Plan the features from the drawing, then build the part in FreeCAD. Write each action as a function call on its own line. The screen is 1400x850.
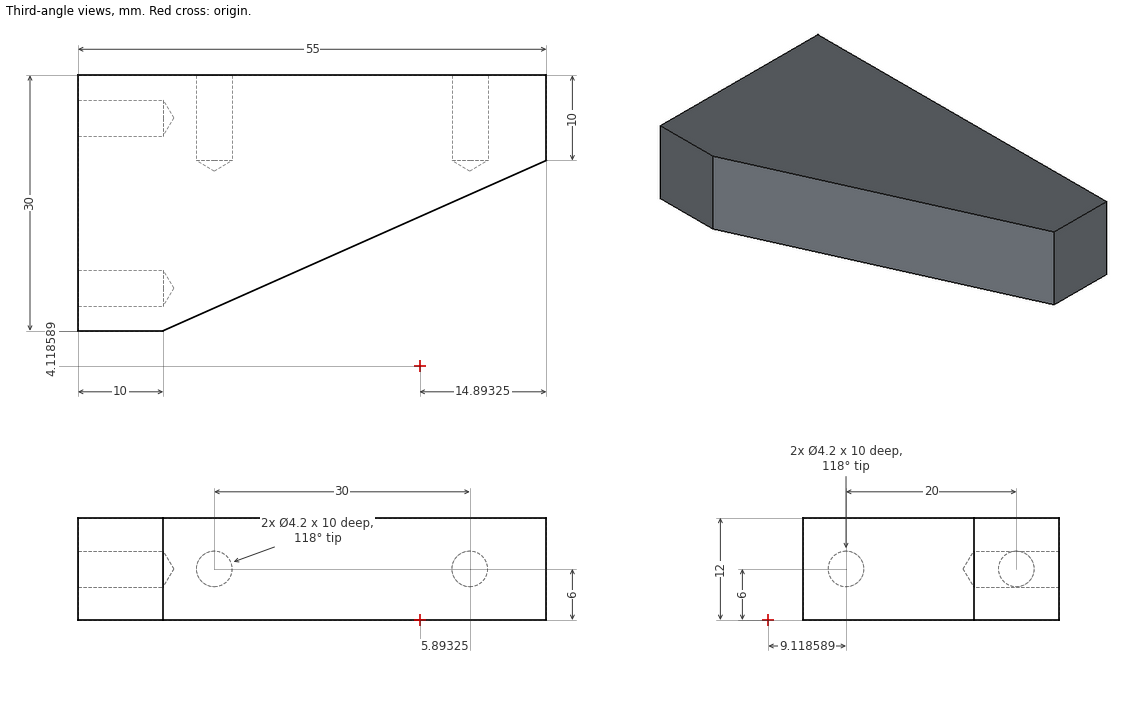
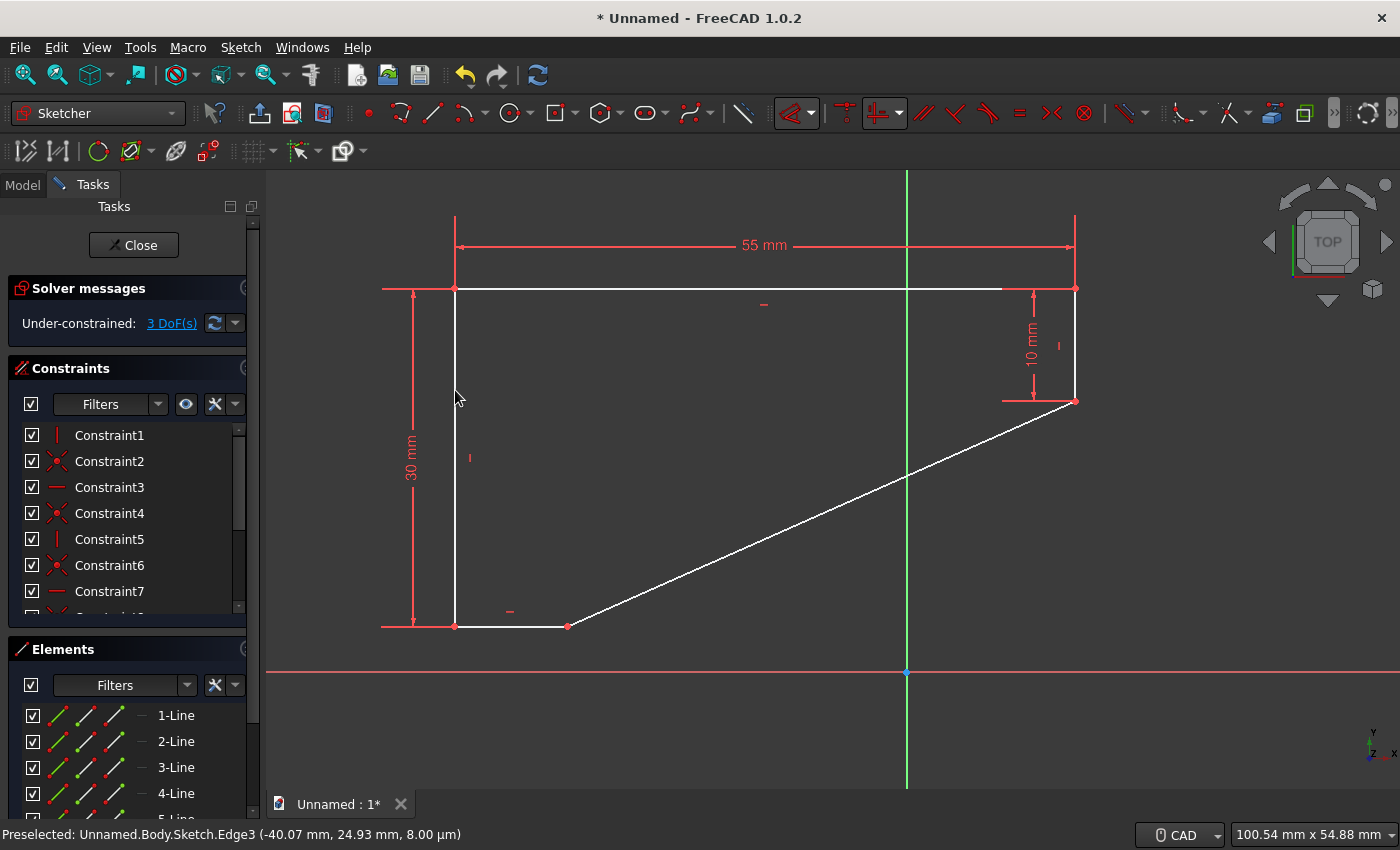
click(488, 627)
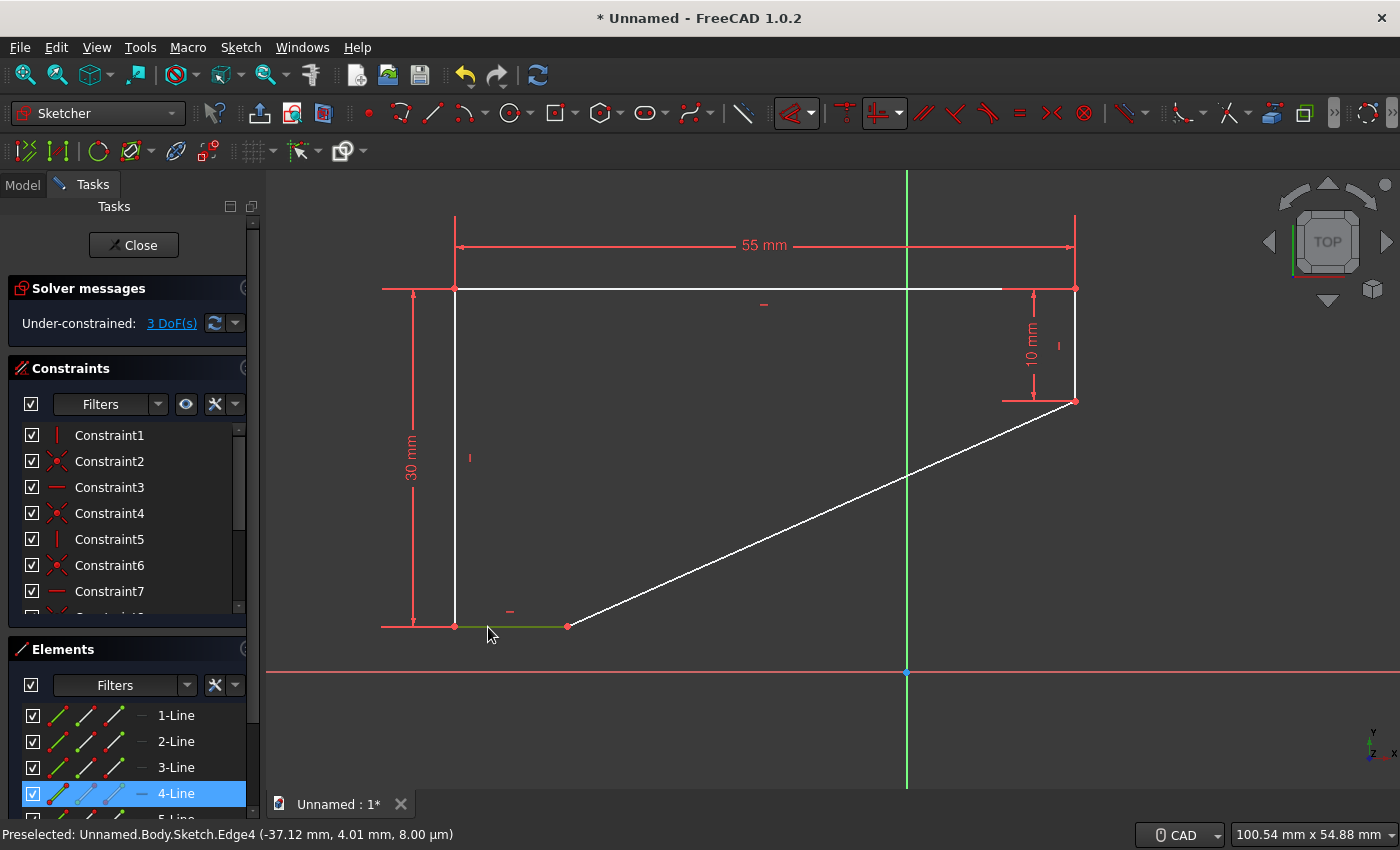
click(814, 114)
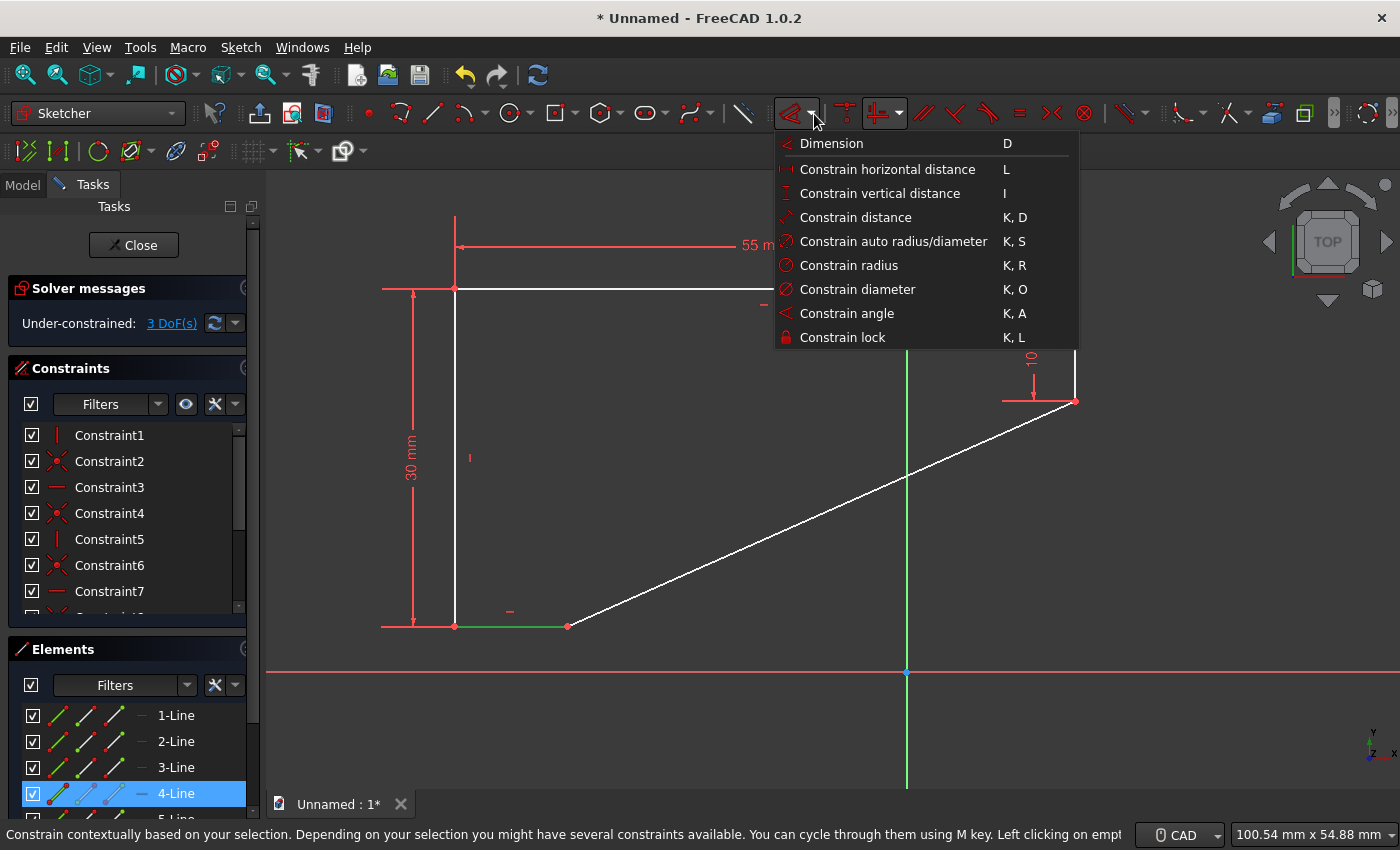
click(927, 169)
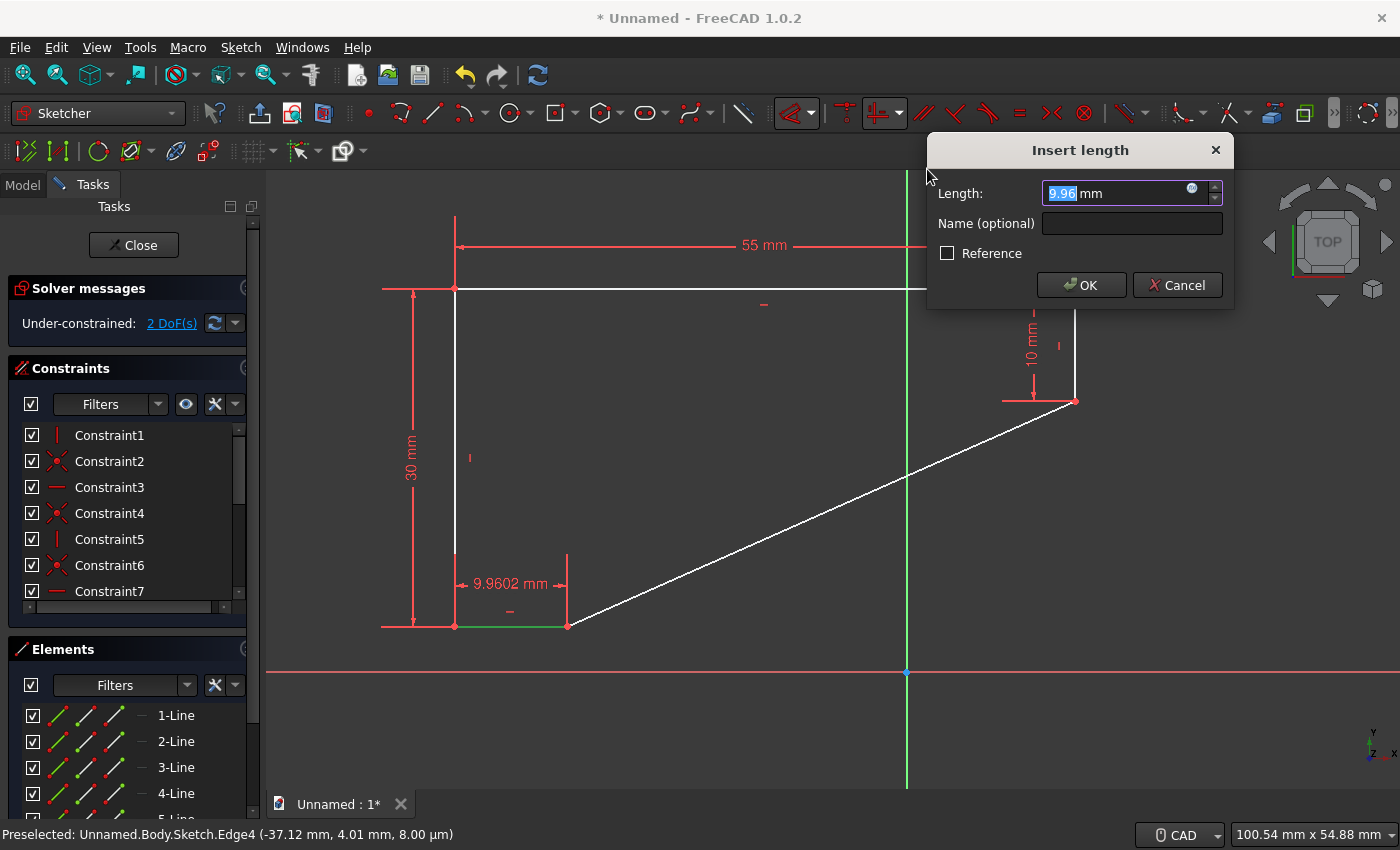
text(10)
key(Return)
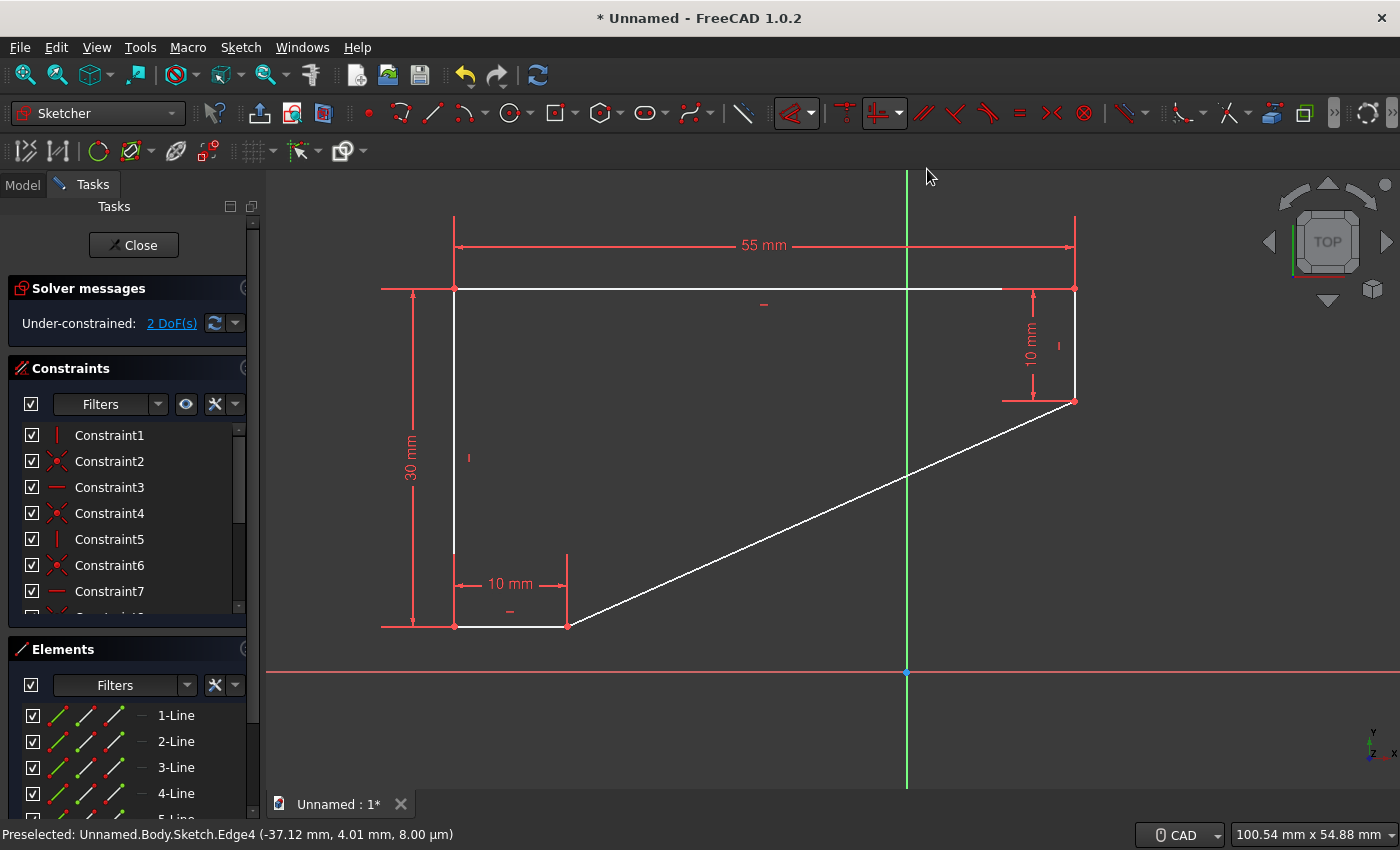
click(1075, 401)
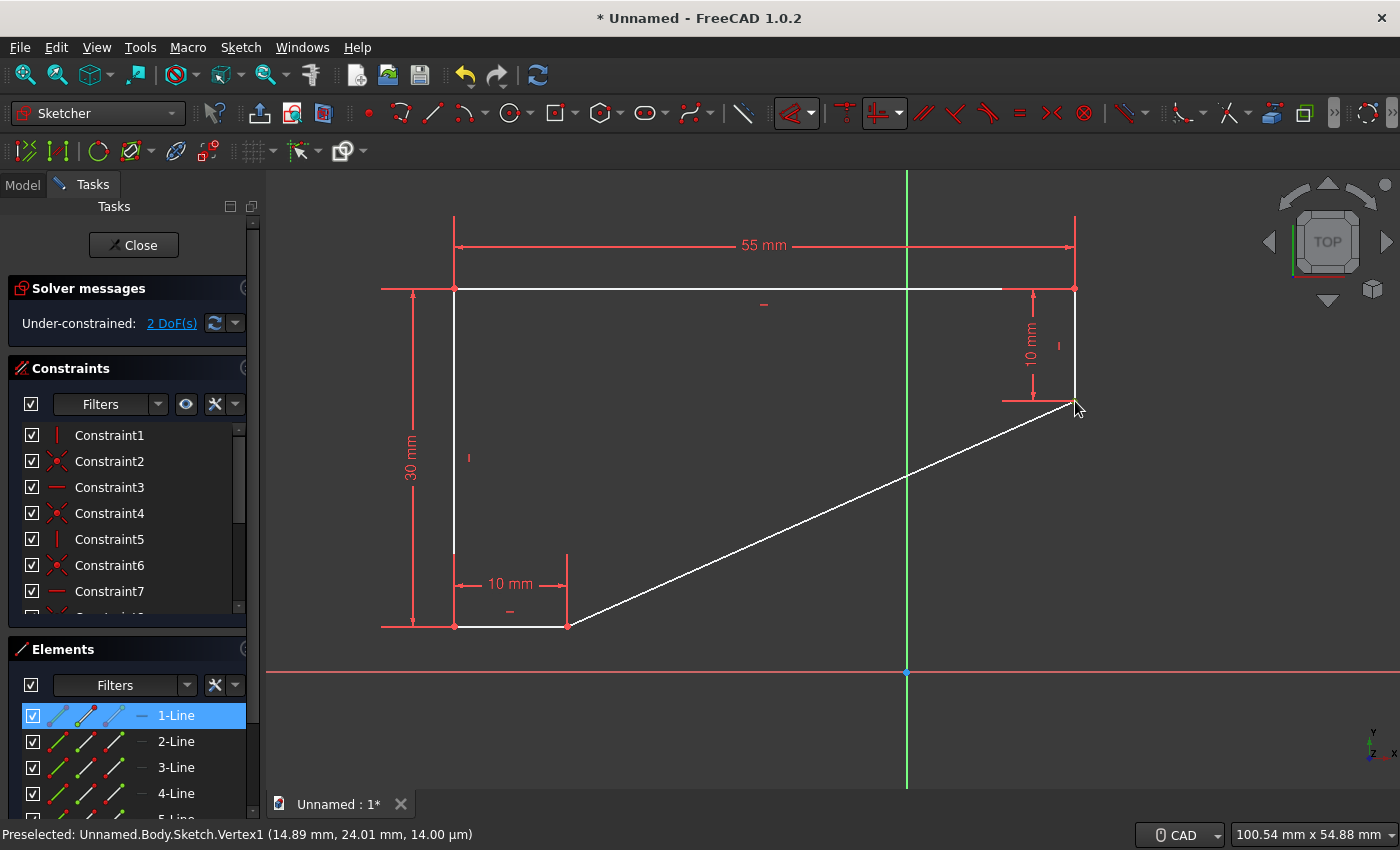
key(l)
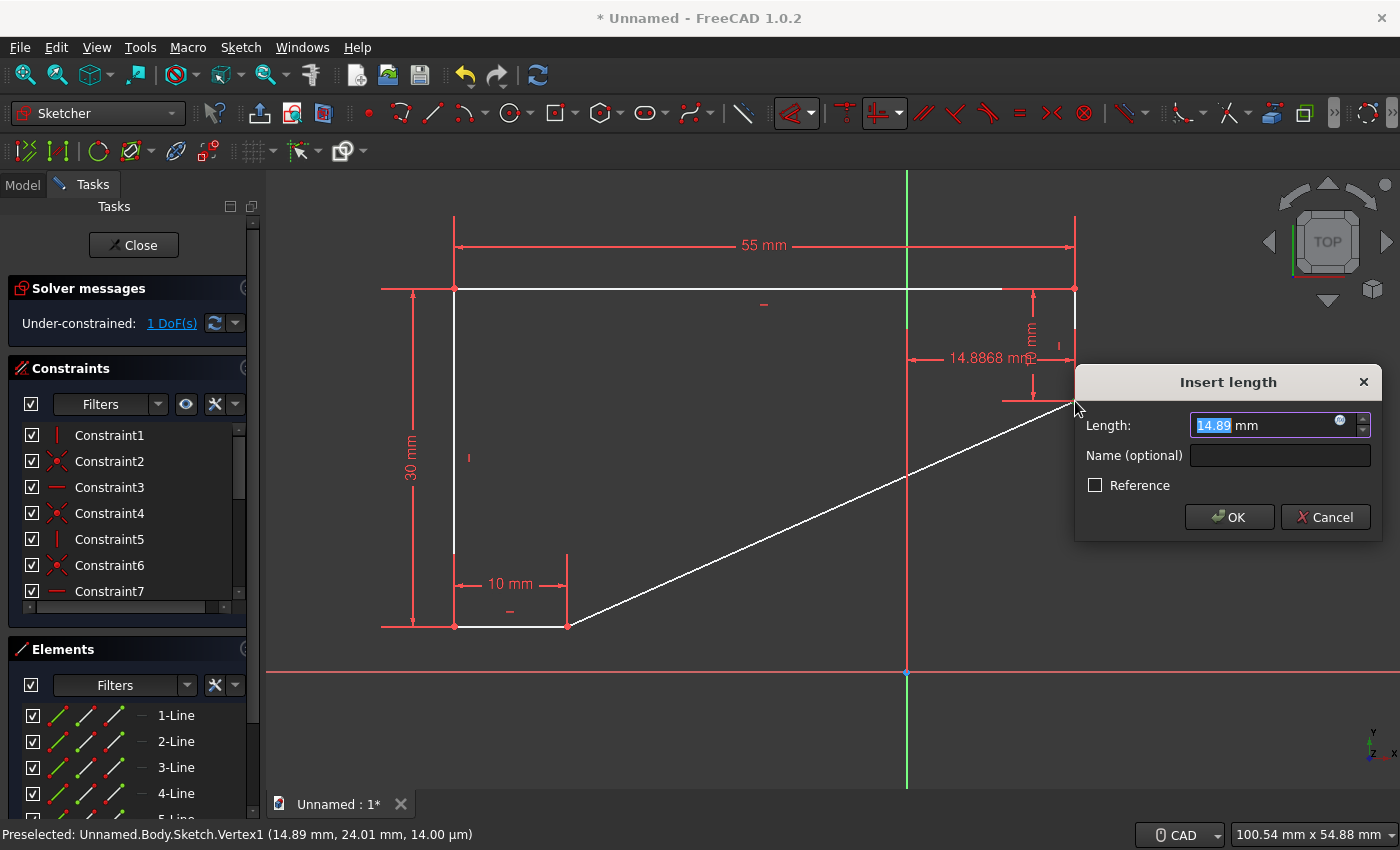
text(14.89325)
key(Return)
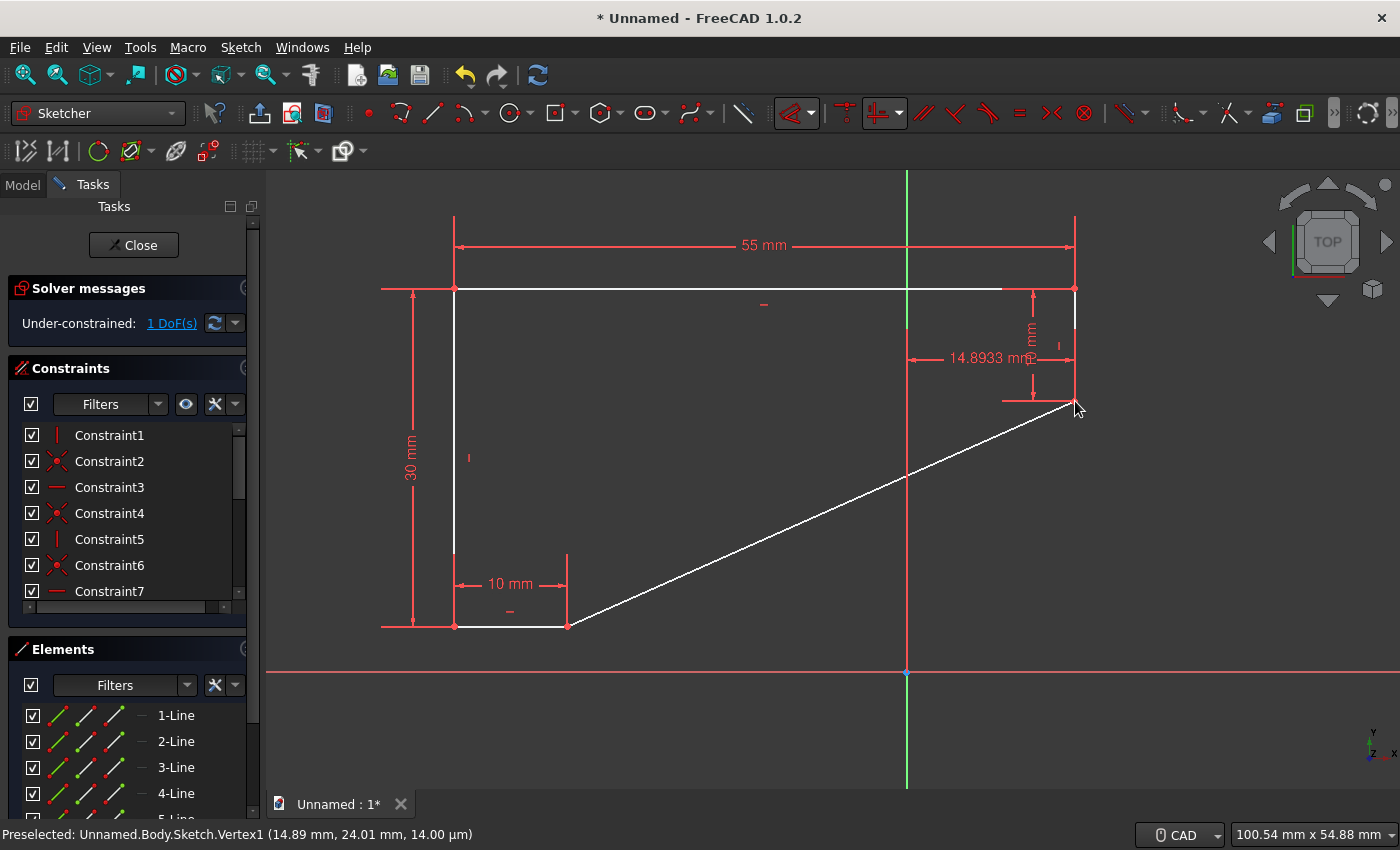
click(454, 627)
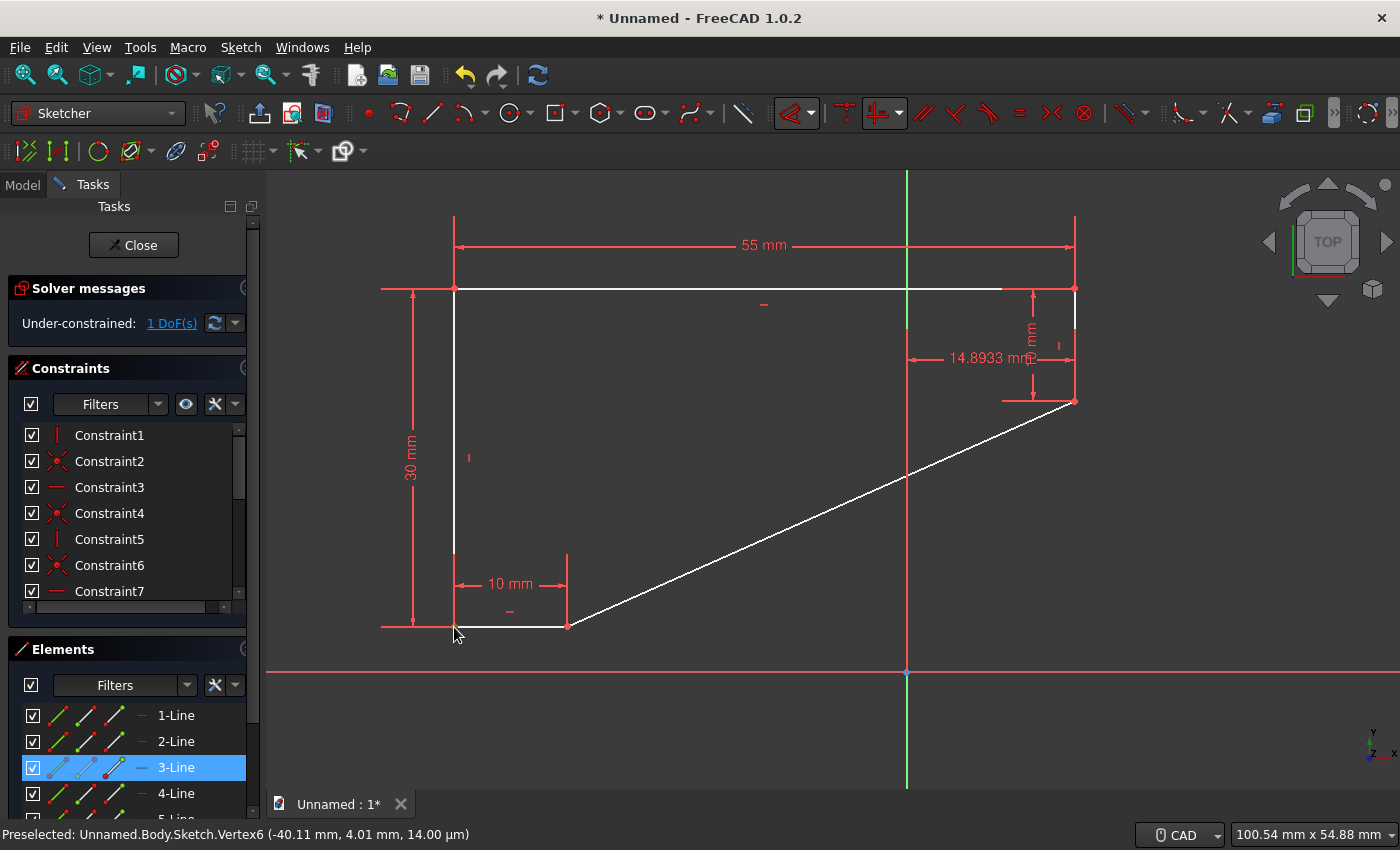
click(814, 114)